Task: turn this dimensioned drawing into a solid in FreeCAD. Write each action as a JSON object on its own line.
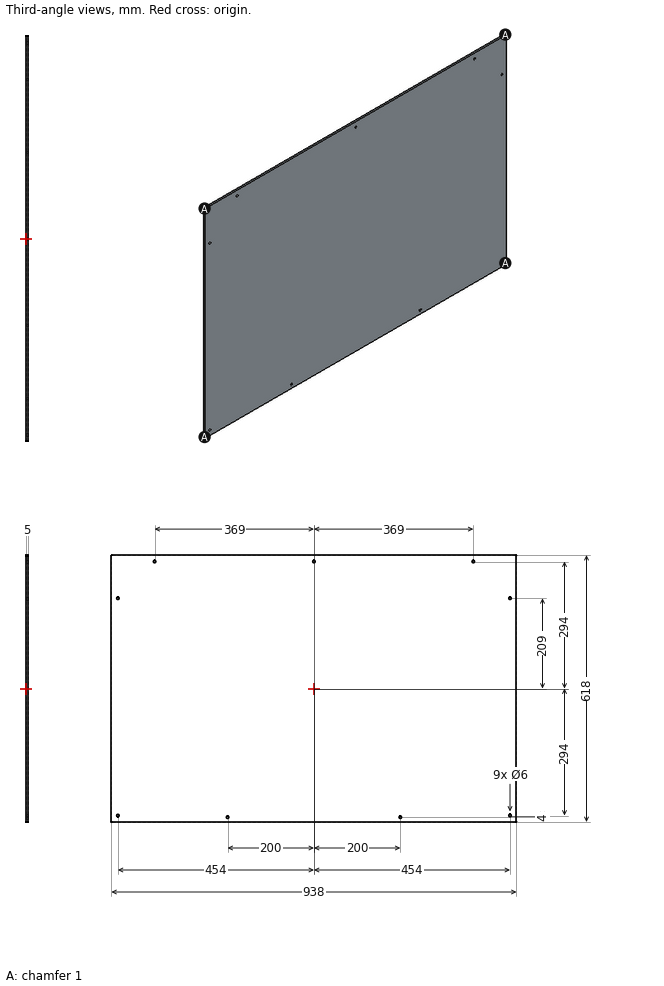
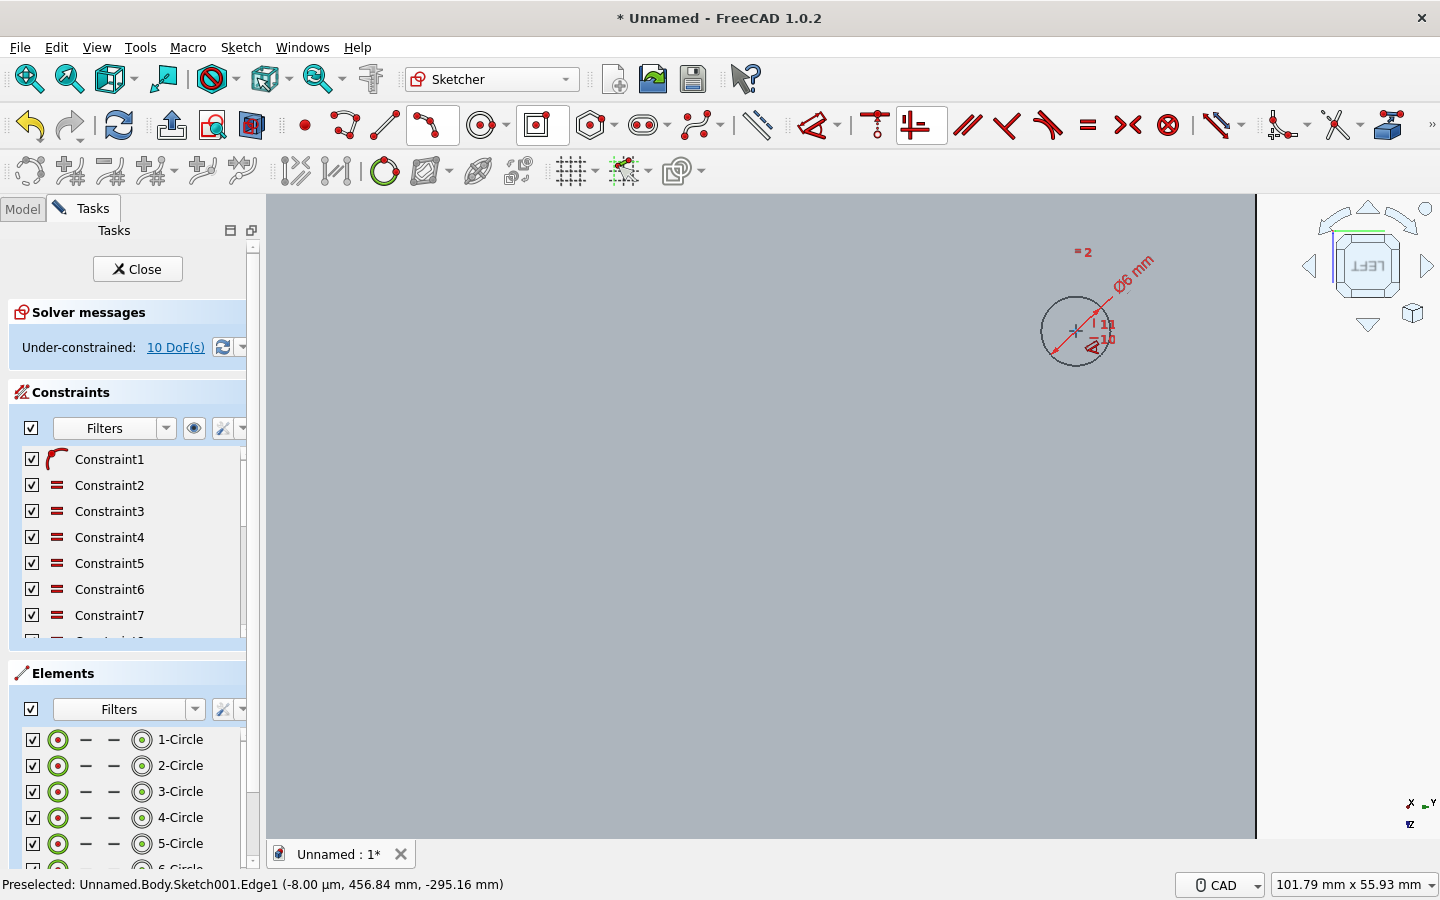
{"action": "left_click", "coordinate": [1076, 331]}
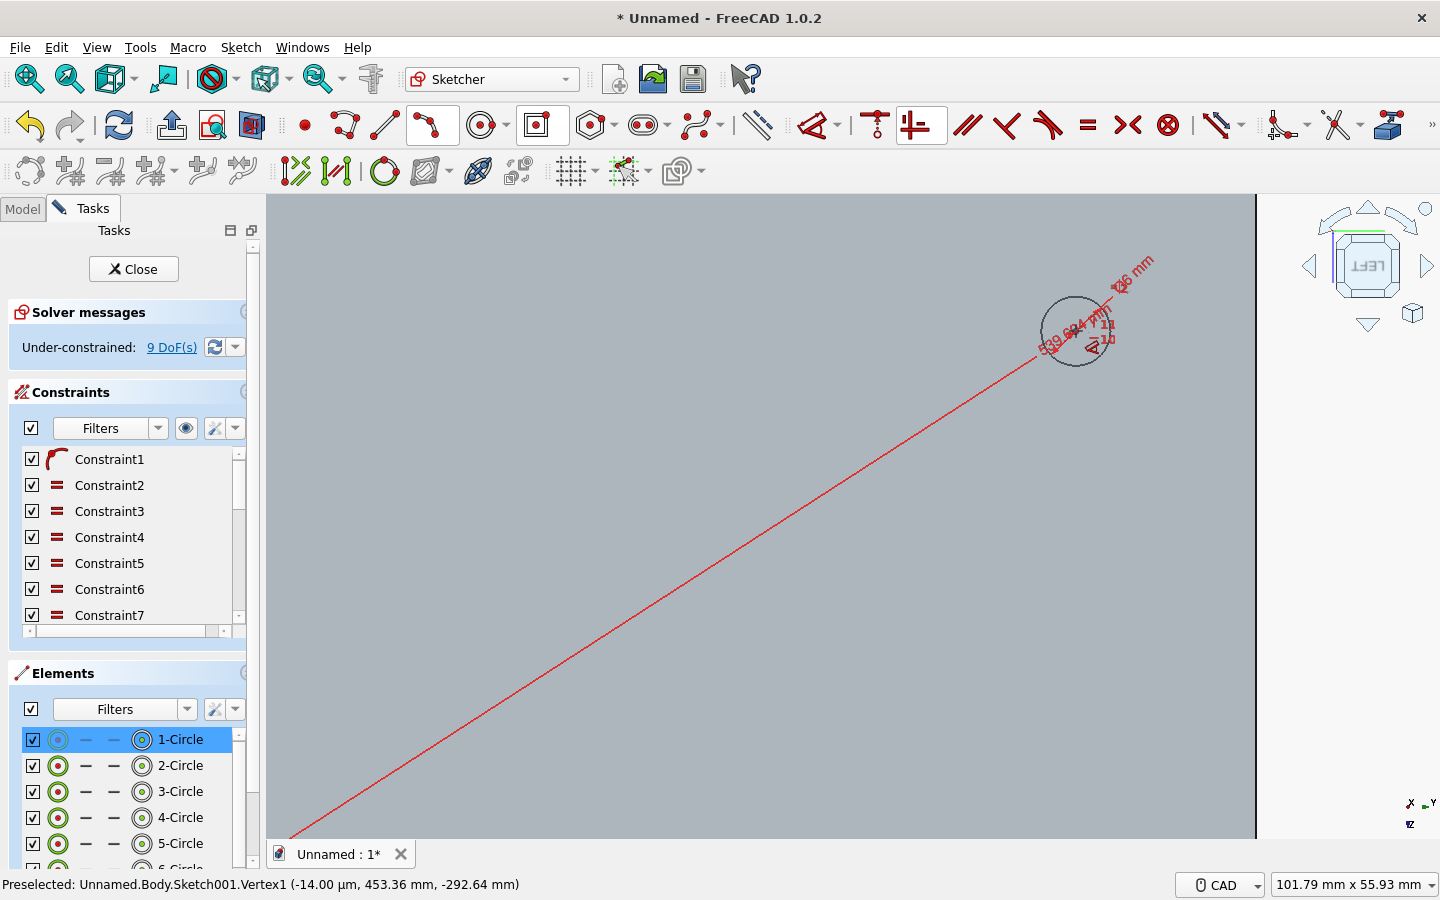
{"action": "scroll", "coordinate": [1104, 311], "scroll_direction": "down", "scroll_amount": 14}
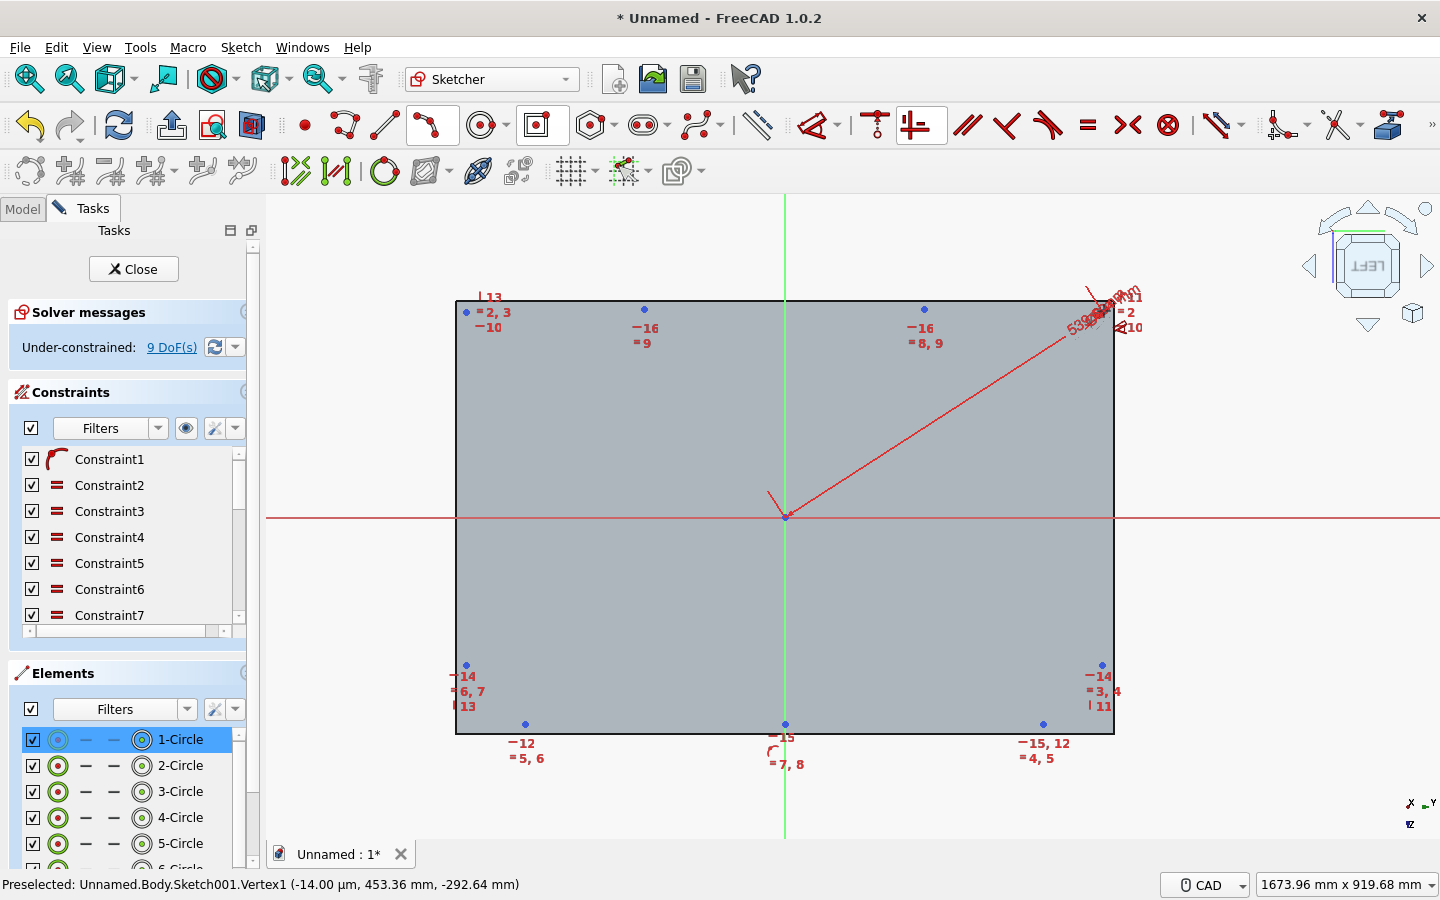
{"action": "scroll", "coordinate": [925, 309], "scroll_direction": "up", "scroll_amount": 14}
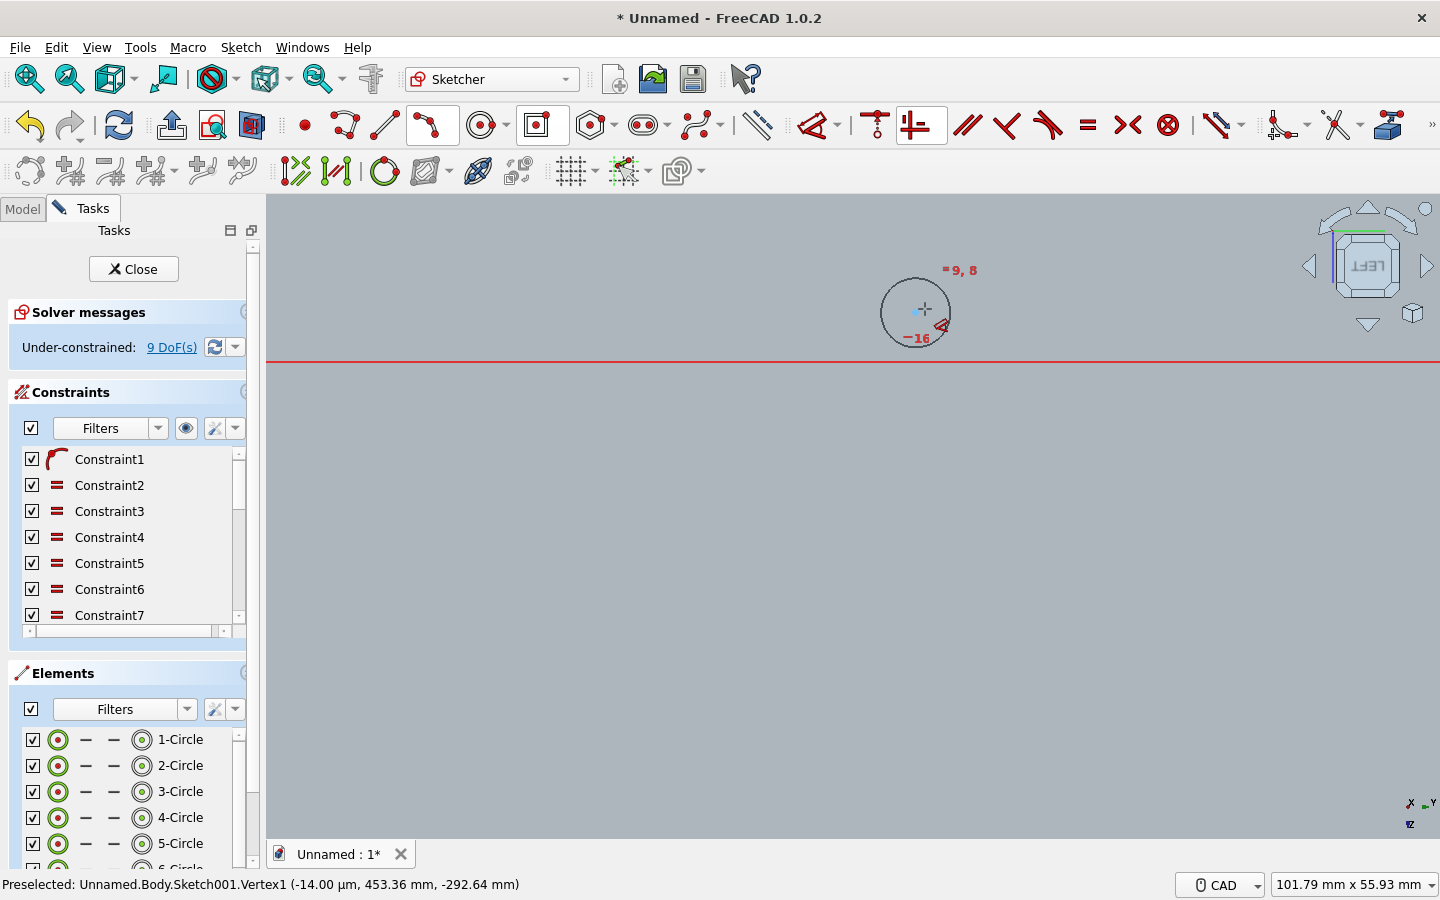
{"action": "left_click", "coordinate": [916, 313]}
{"action": "left_click", "coordinate": [882, 349]}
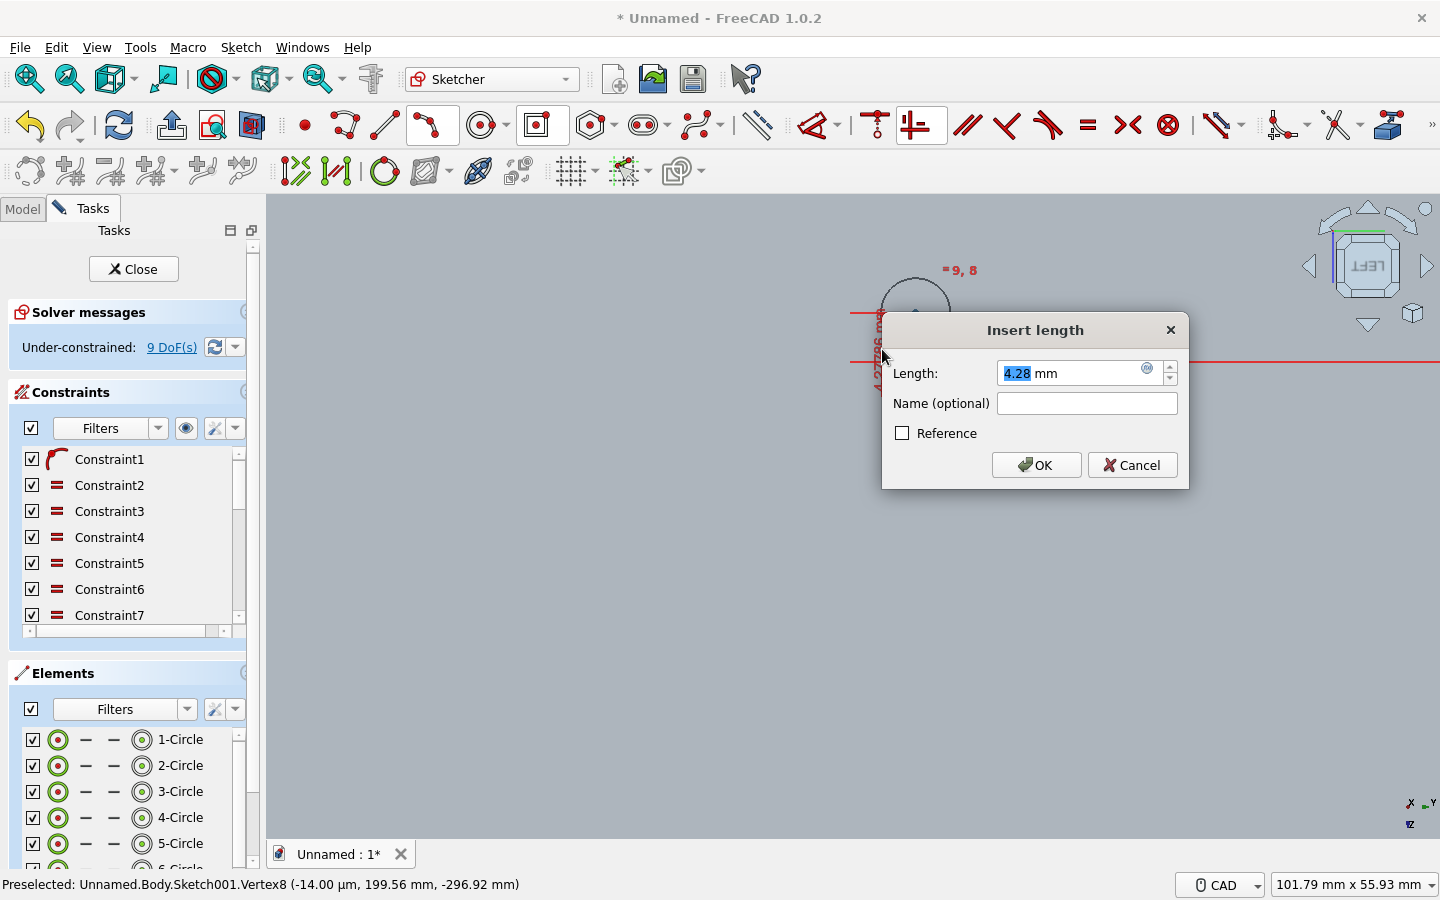
{"action": "type", "text": "4"}
{"action": "key", "text": "Return"}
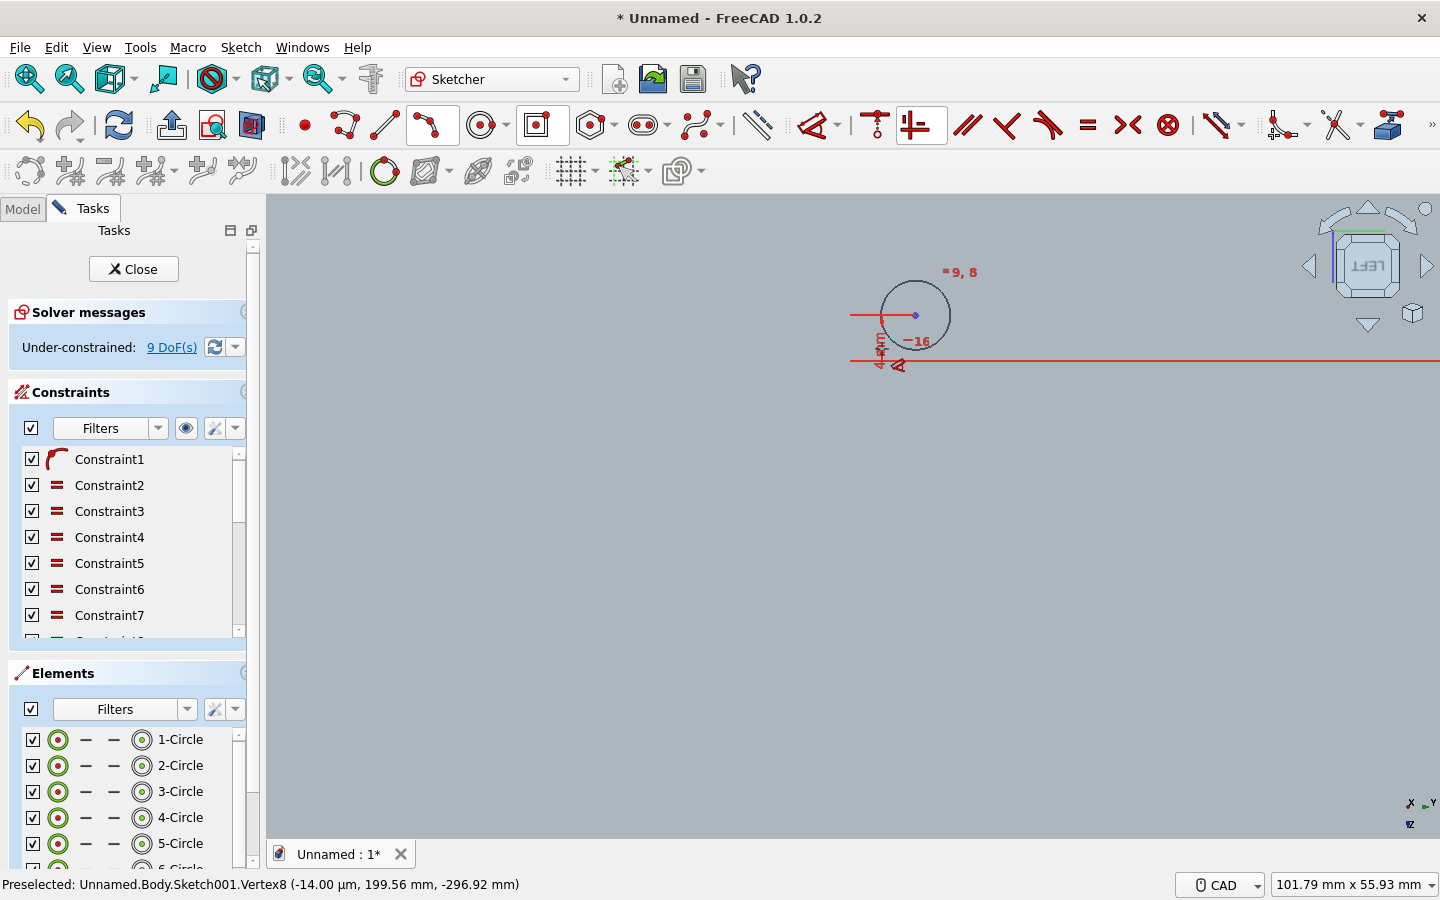
{"action": "scroll", "coordinate": [925, 309], "scroll_direction": "down", "scroll_amount": 14}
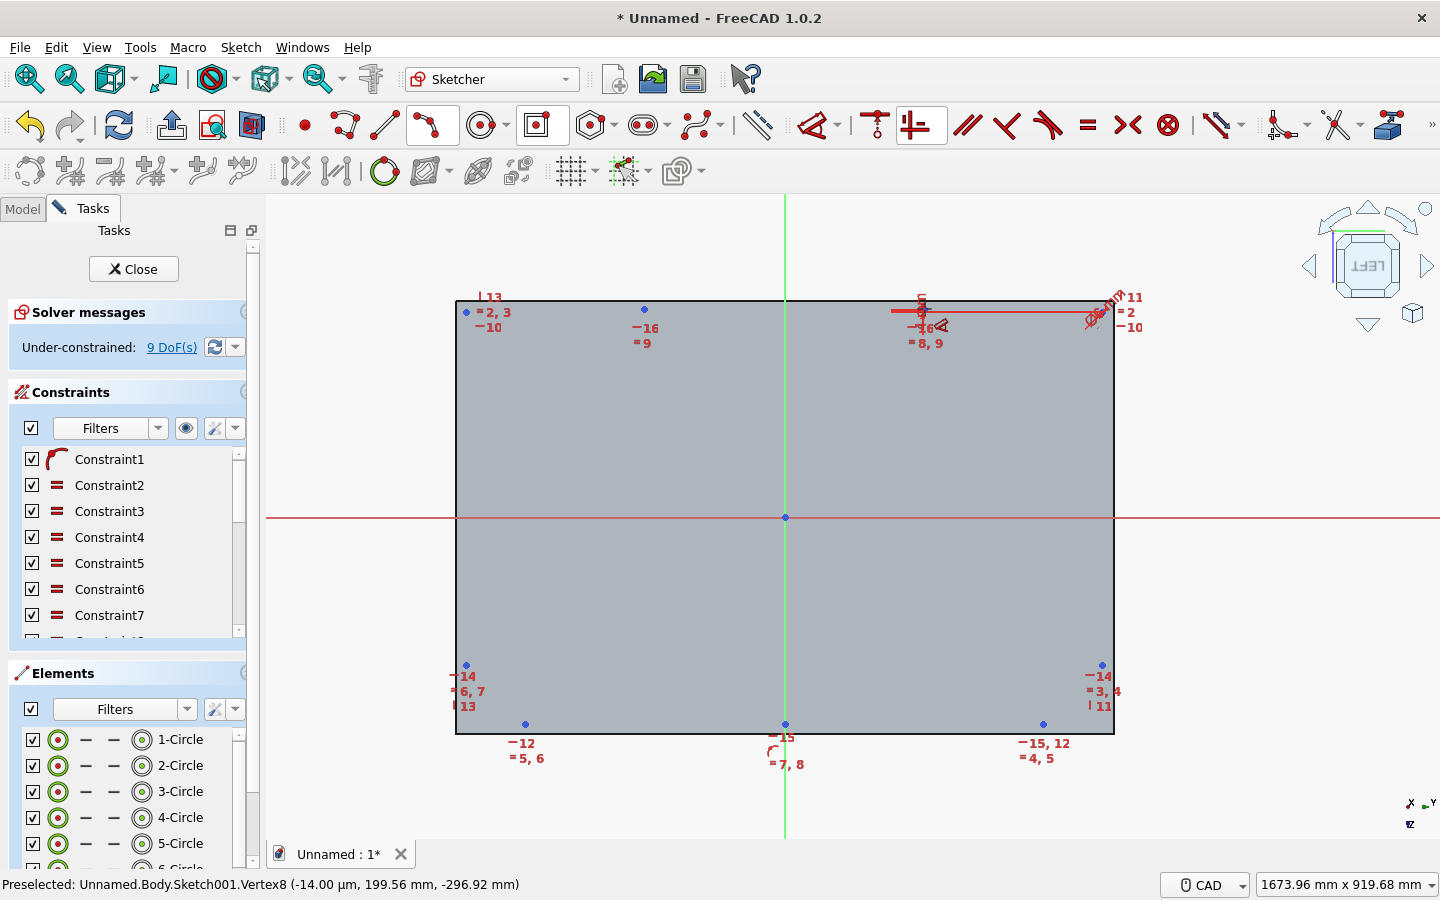
{"action": "left_click", "coordinate": [1103, 312]}
{"action": "left_click", "coordinate": [944, 278]}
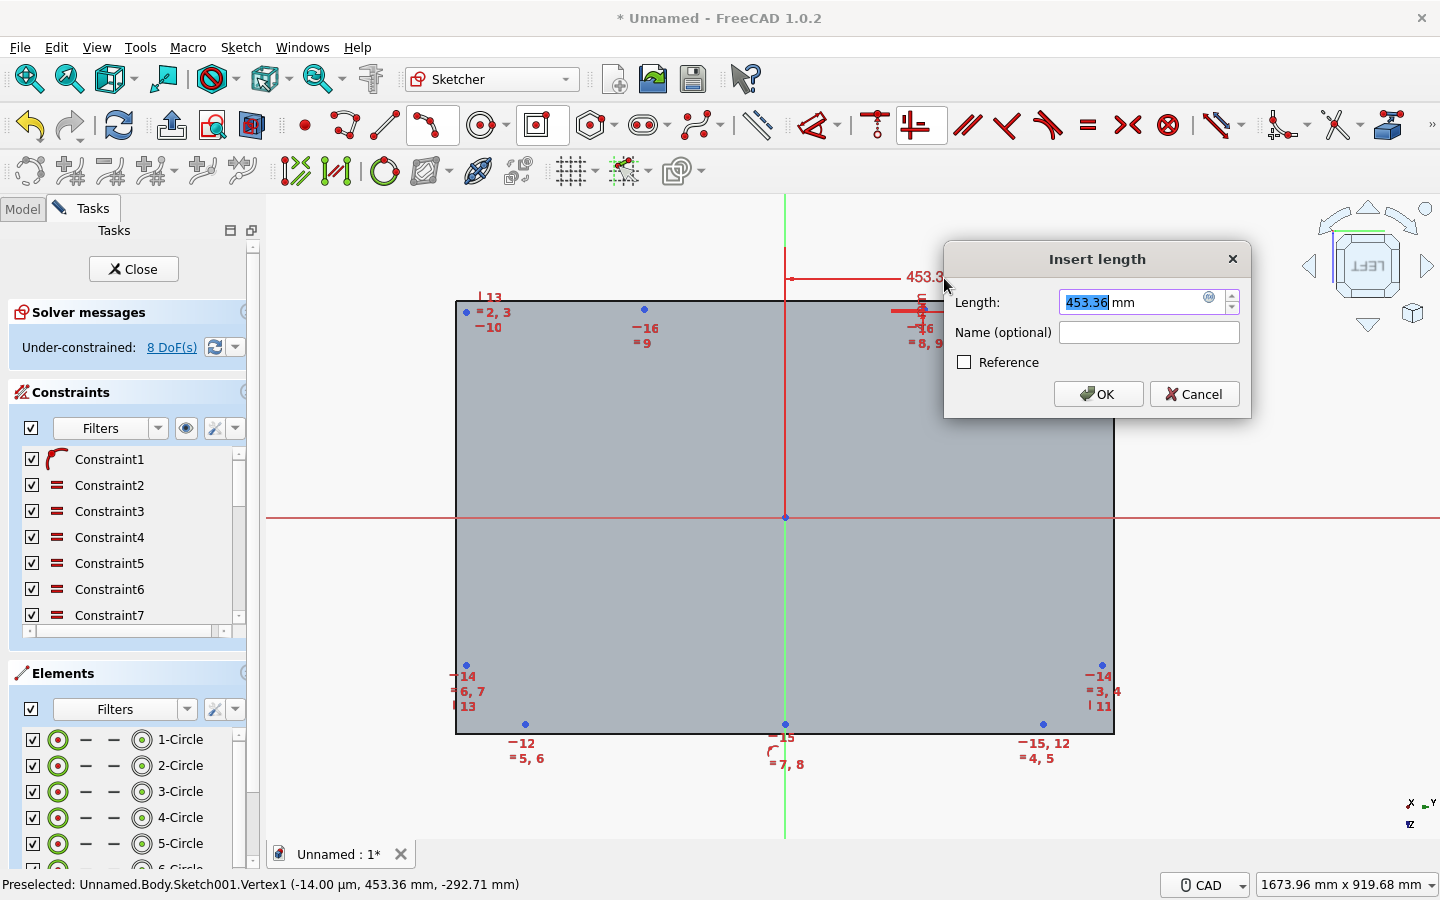
{"action": "type", "text": "454"}
{"action": "key", "text": "Return"}